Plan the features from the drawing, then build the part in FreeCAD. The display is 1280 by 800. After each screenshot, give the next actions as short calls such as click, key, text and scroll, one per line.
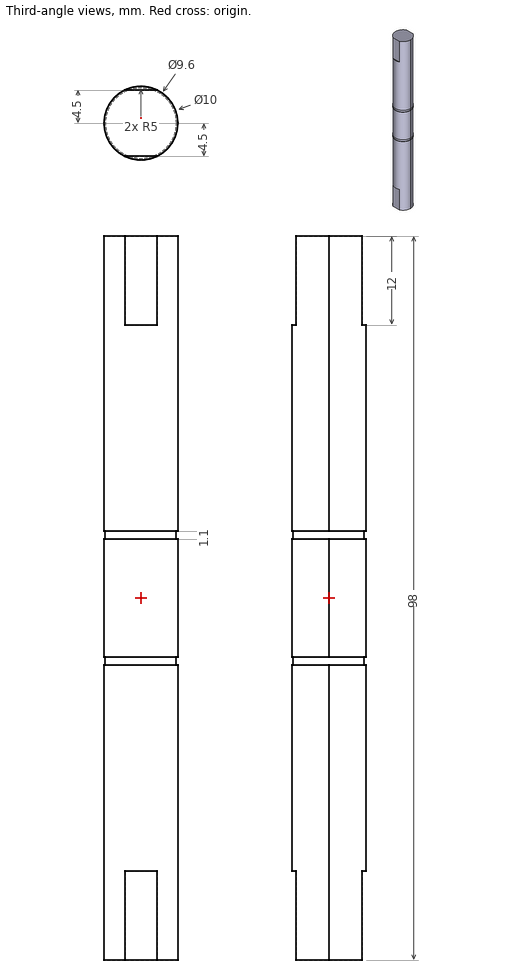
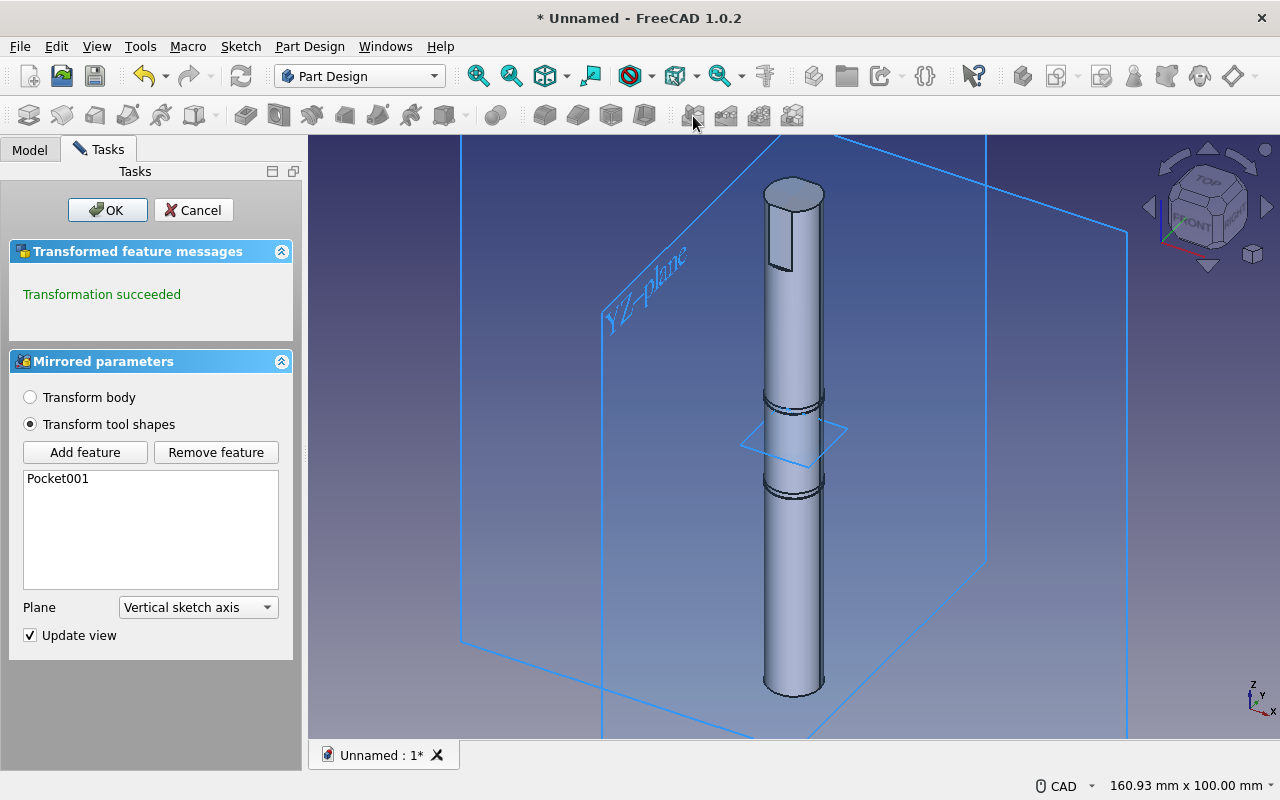
click(199, 608)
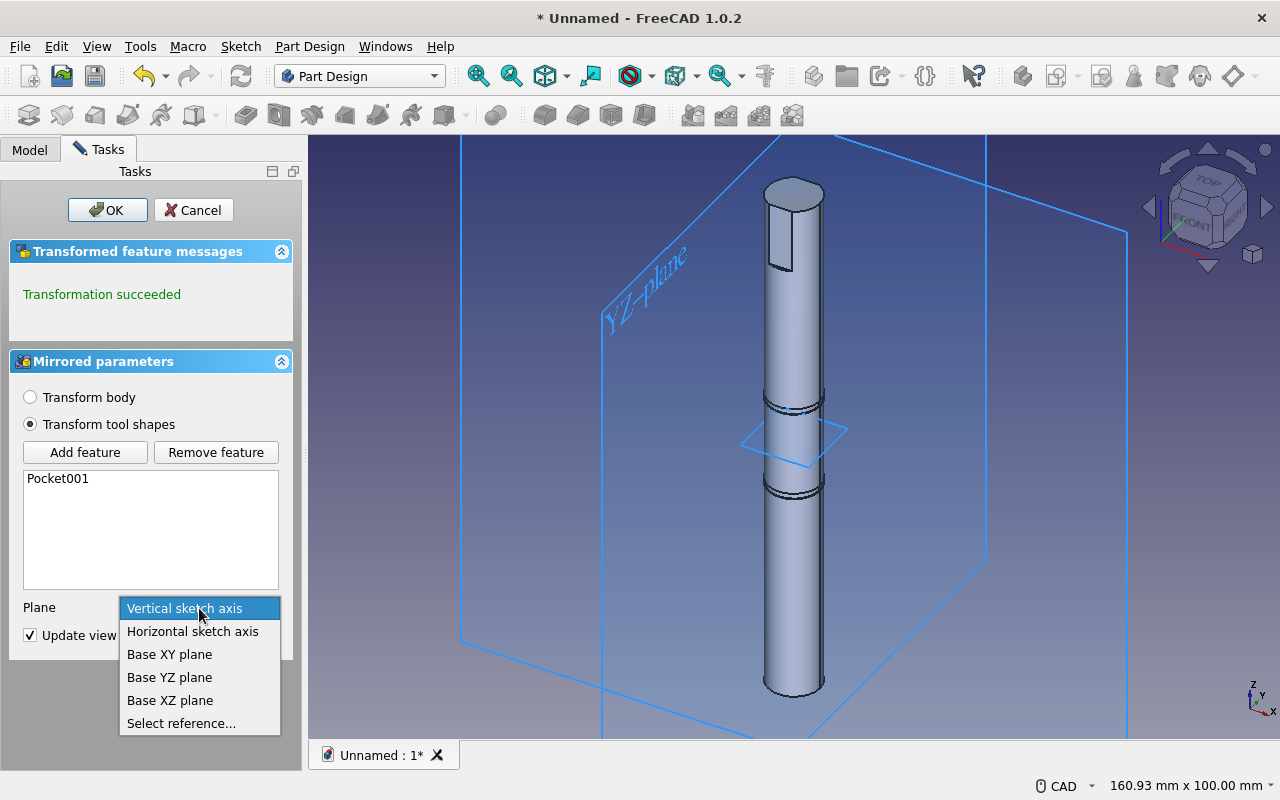
click(198, 654)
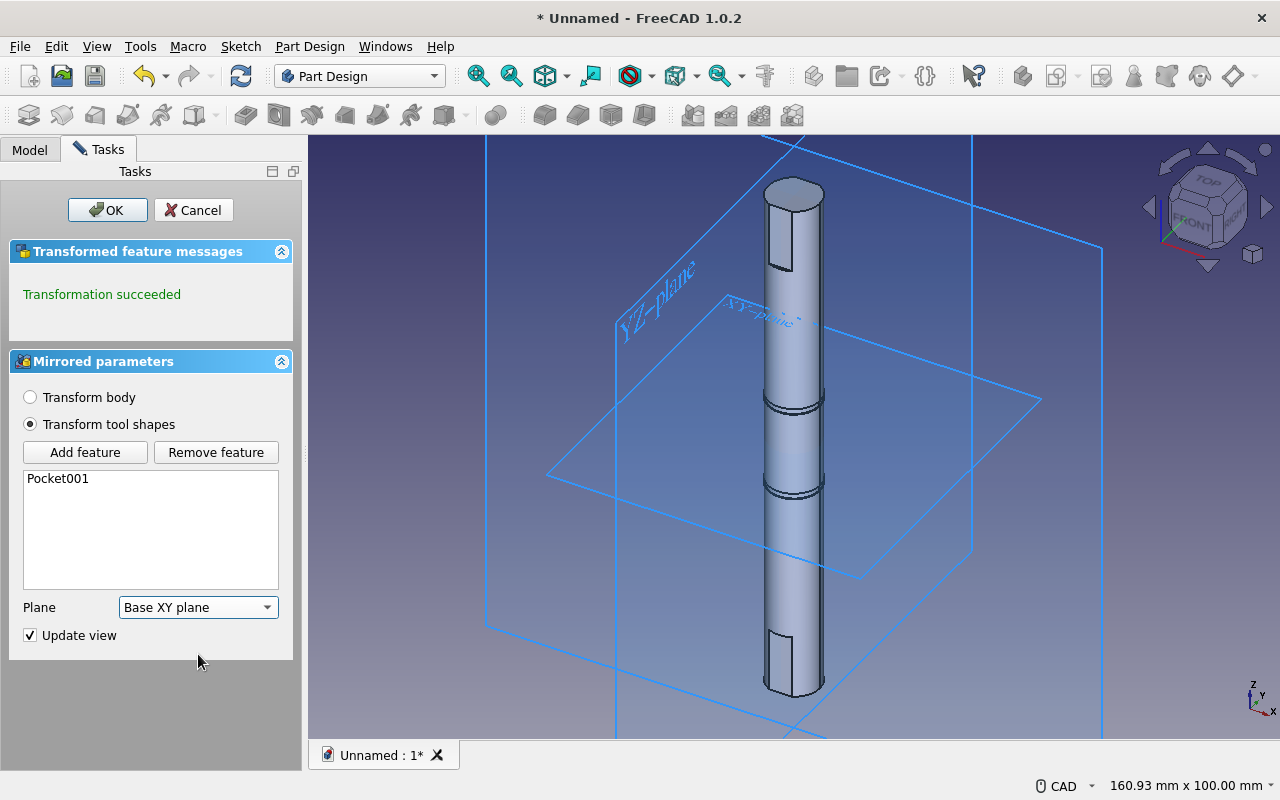
click(108, 210)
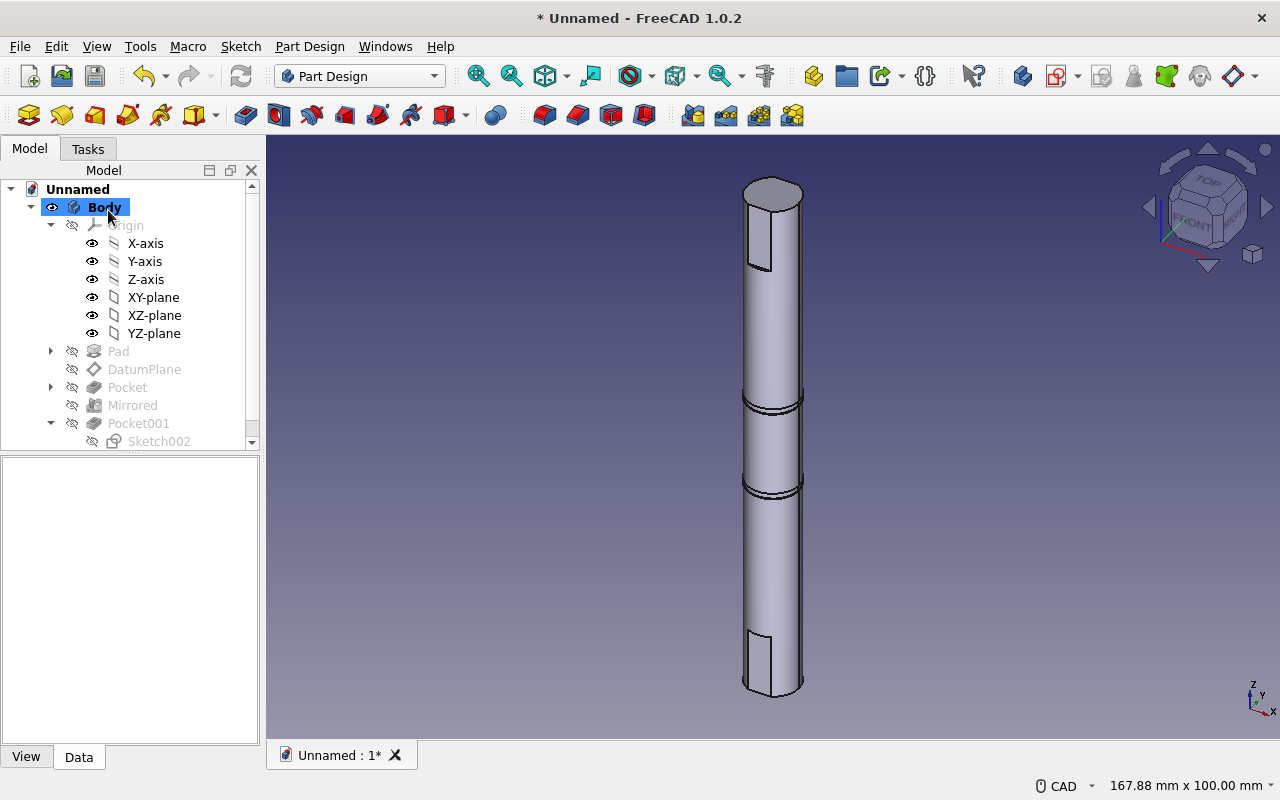
key(0)